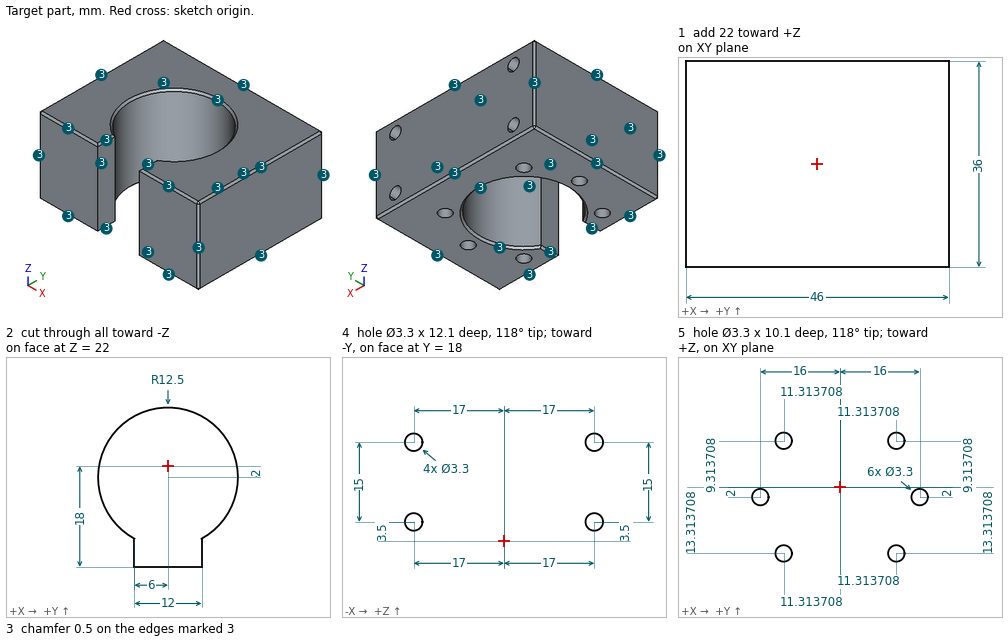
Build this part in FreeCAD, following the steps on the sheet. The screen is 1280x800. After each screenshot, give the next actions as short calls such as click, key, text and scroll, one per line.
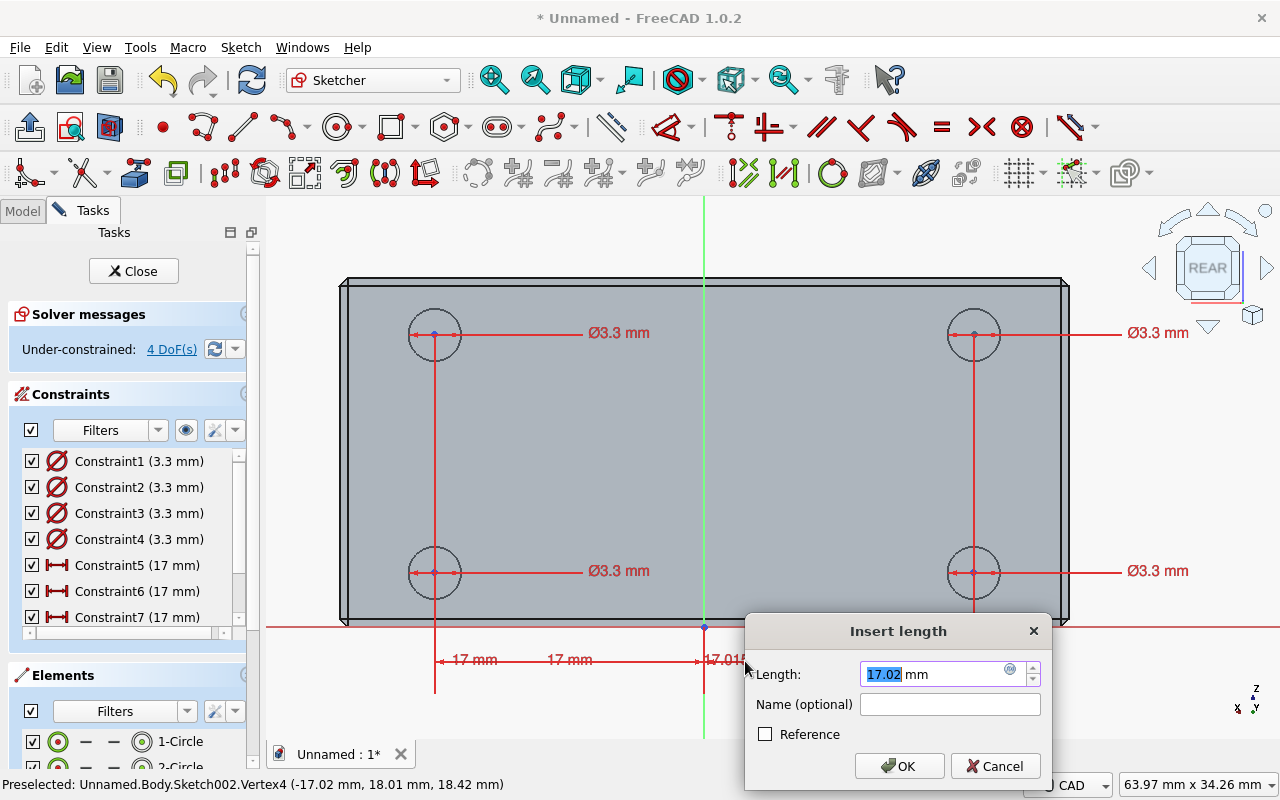
text(17)
key(Return)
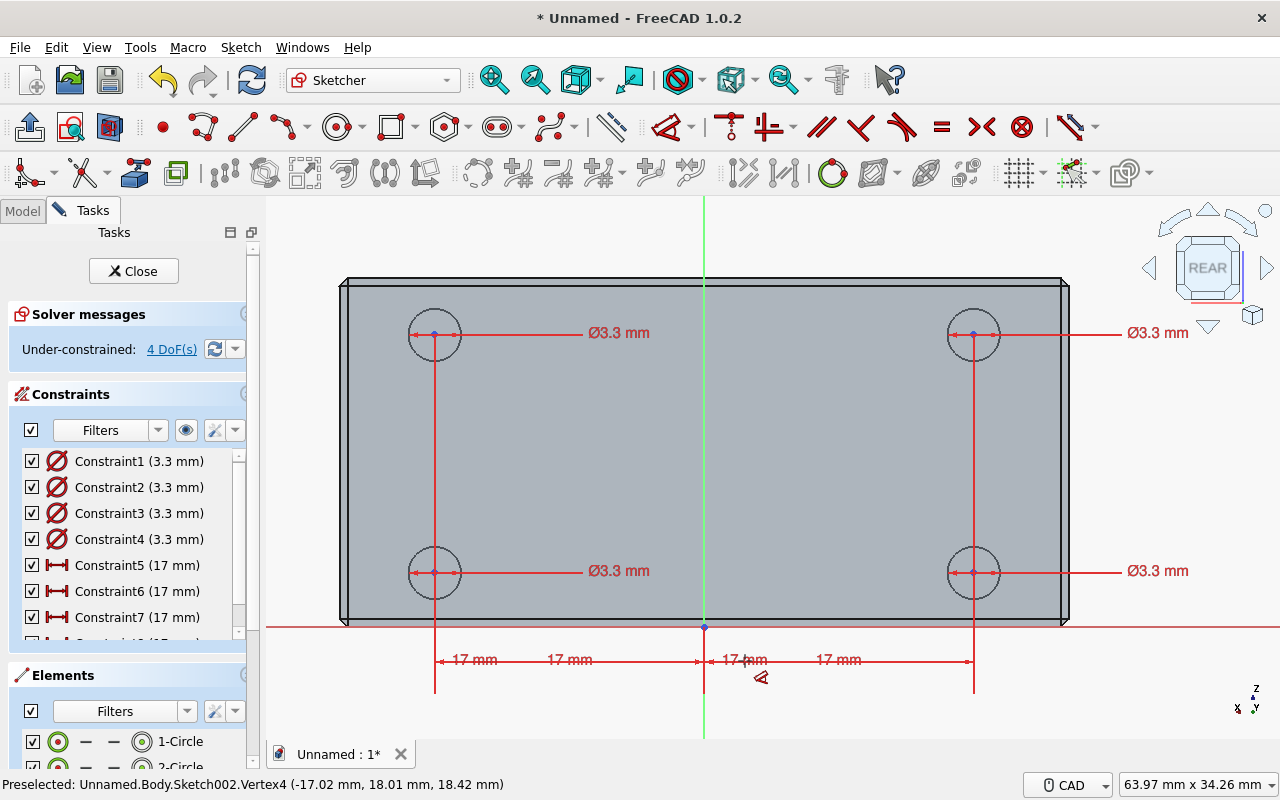
click(435, 573)
click(401, 600)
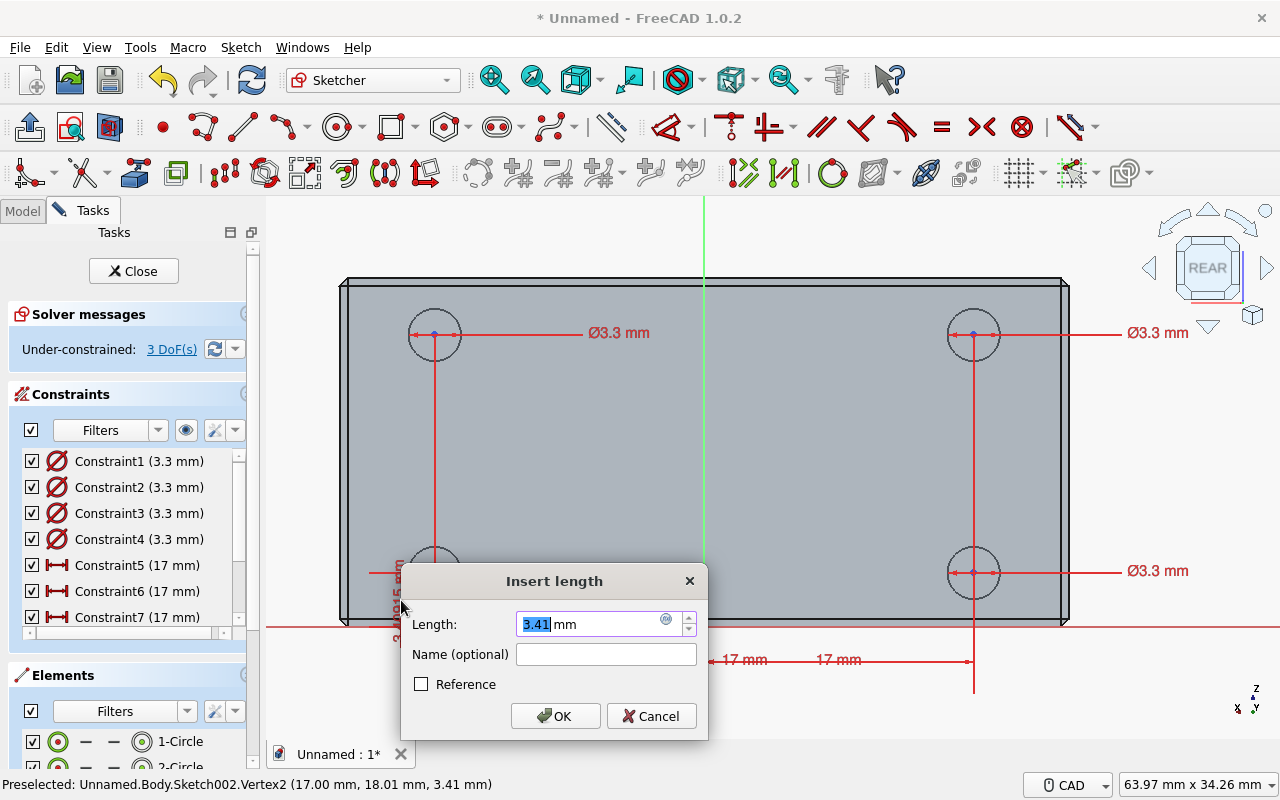
text(3.5)
key(Return)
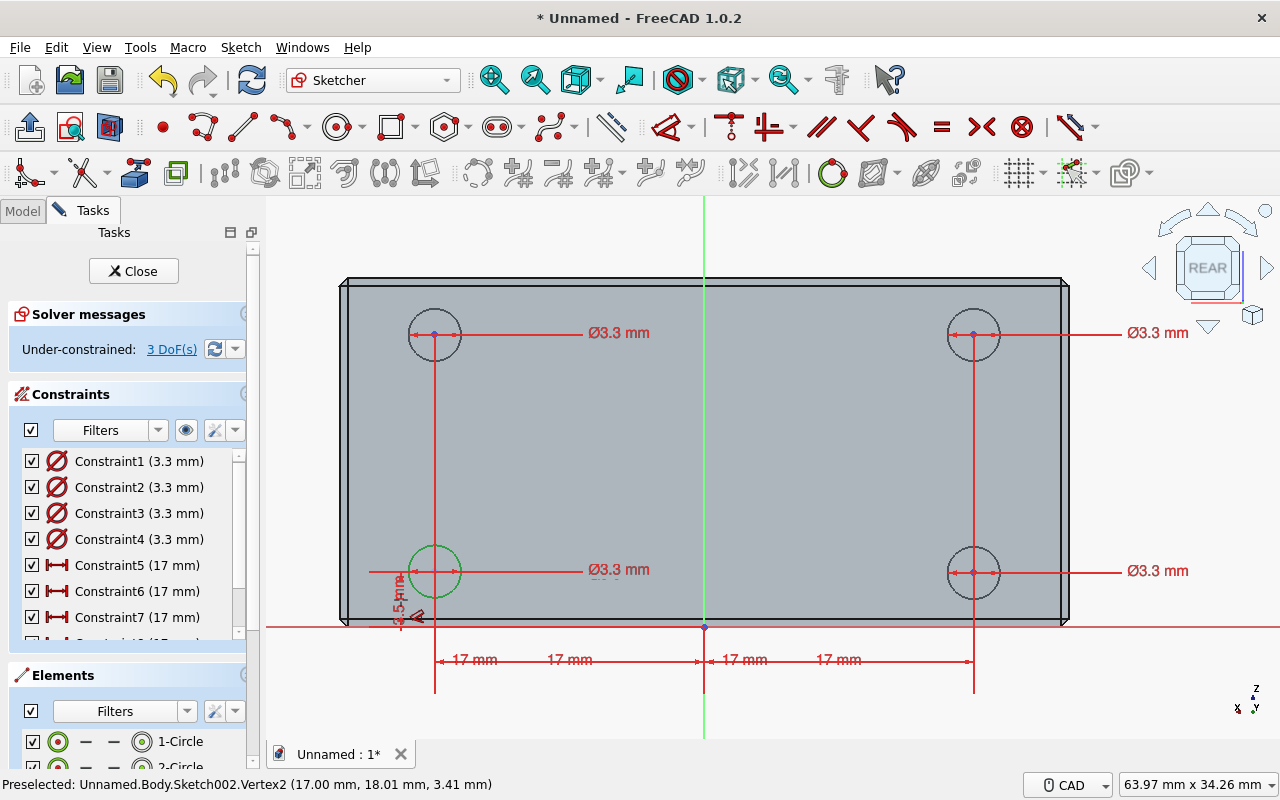
click(974, 573)
click(1008, 600)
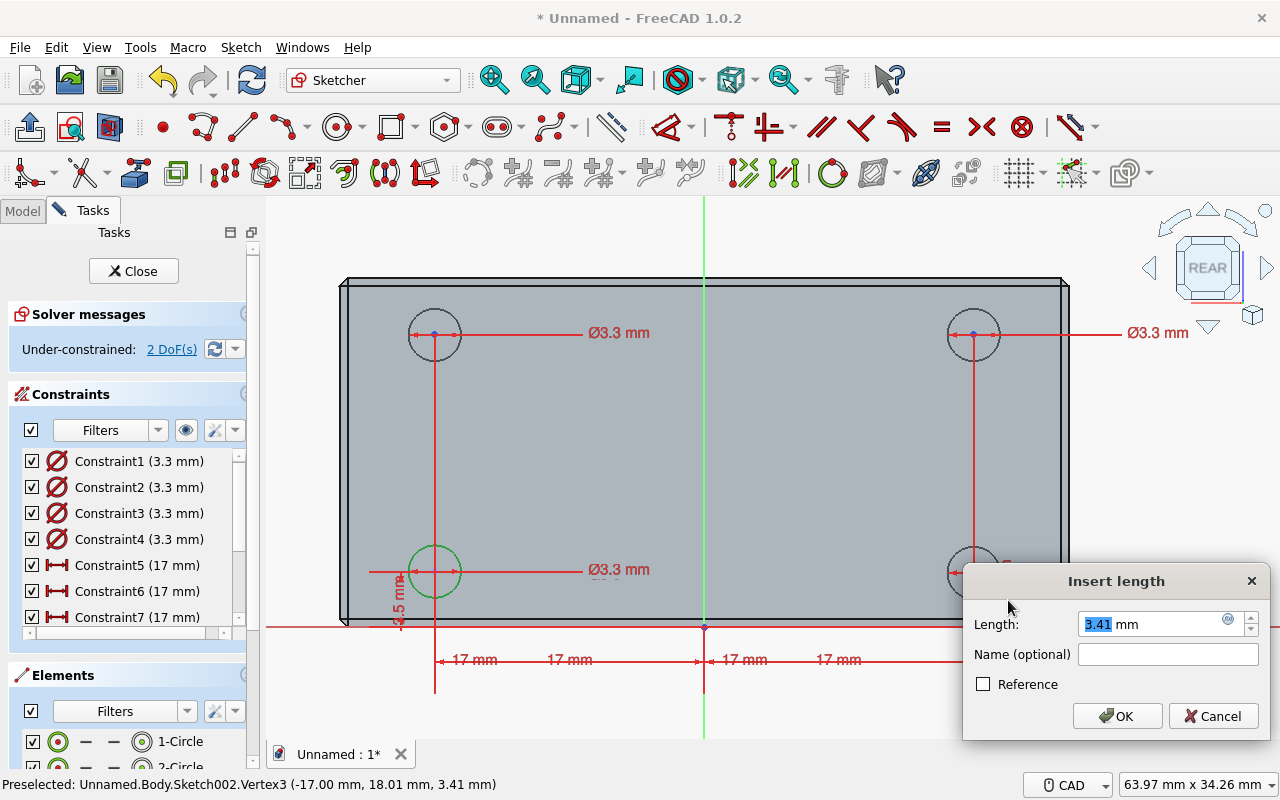
text(3.5)
key(Return)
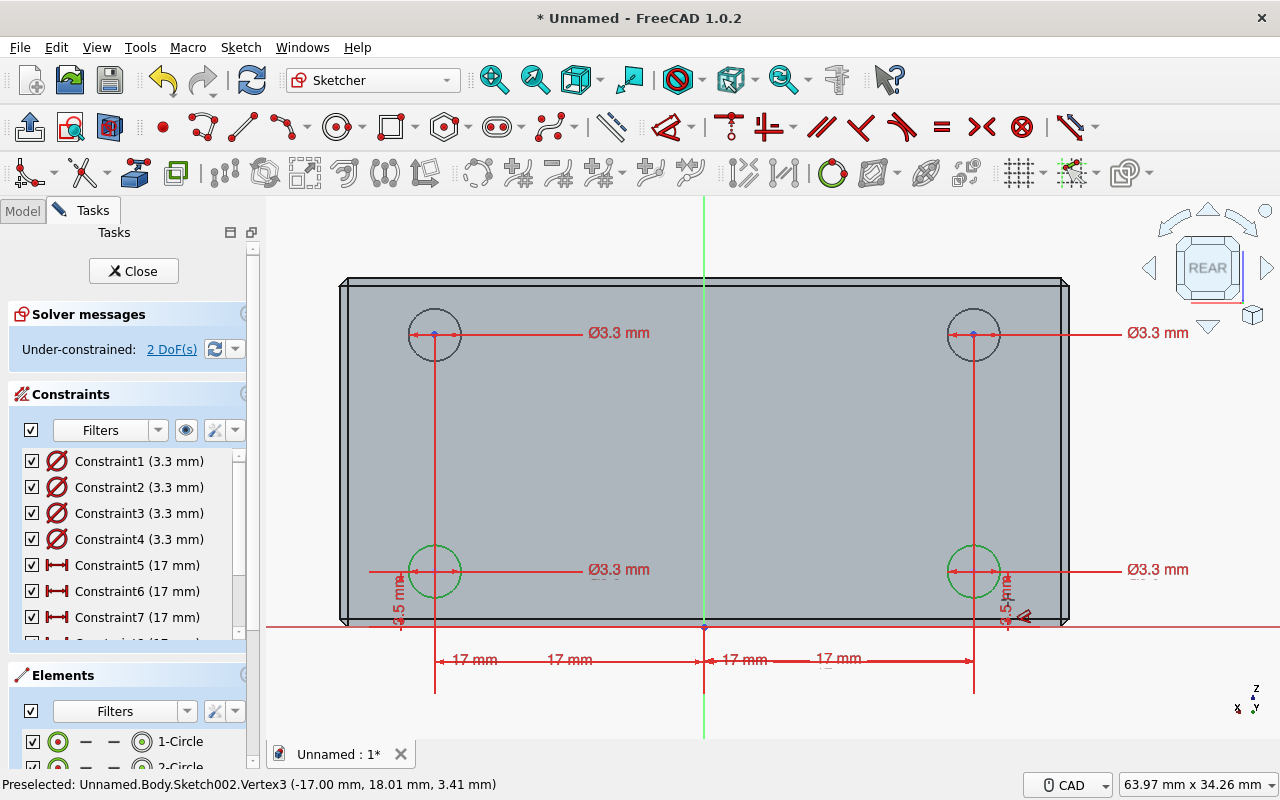
click(435, 335)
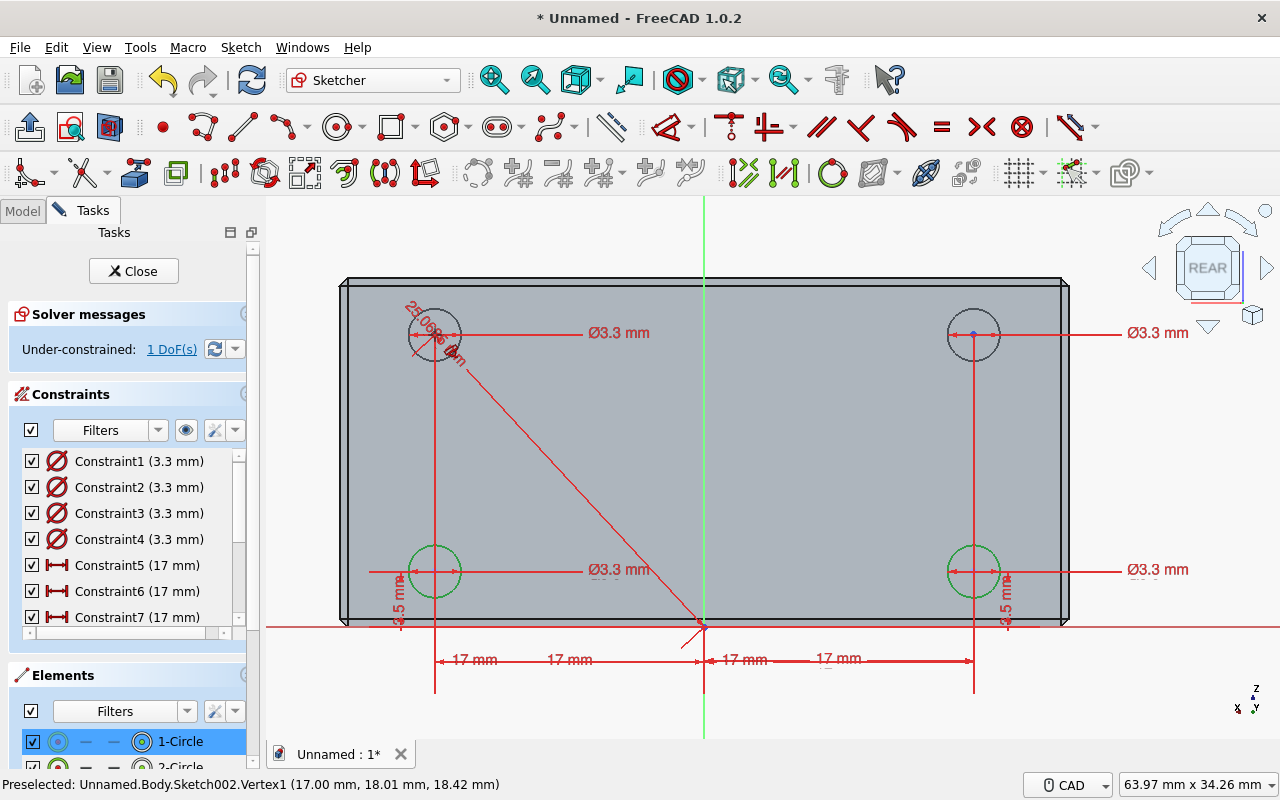
click(435, 572)
click(401, 453)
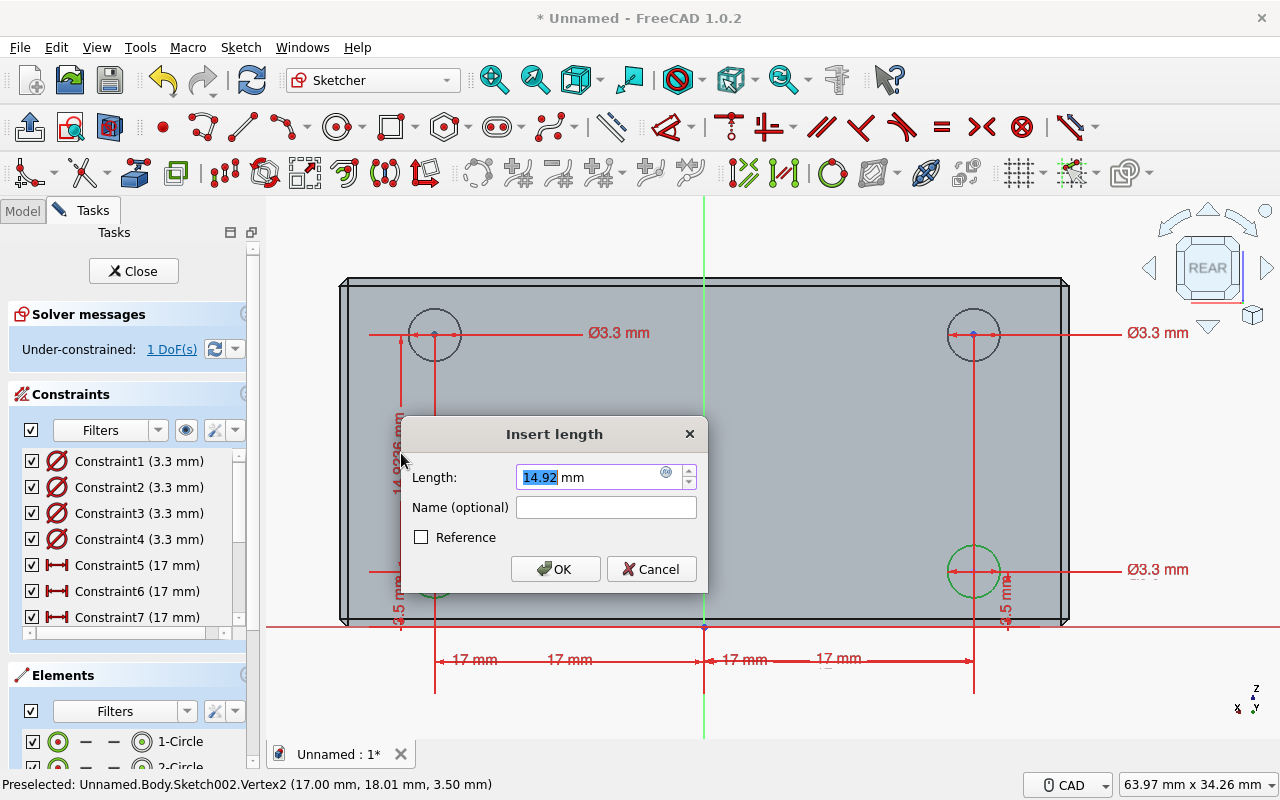
text(15)
key(Return)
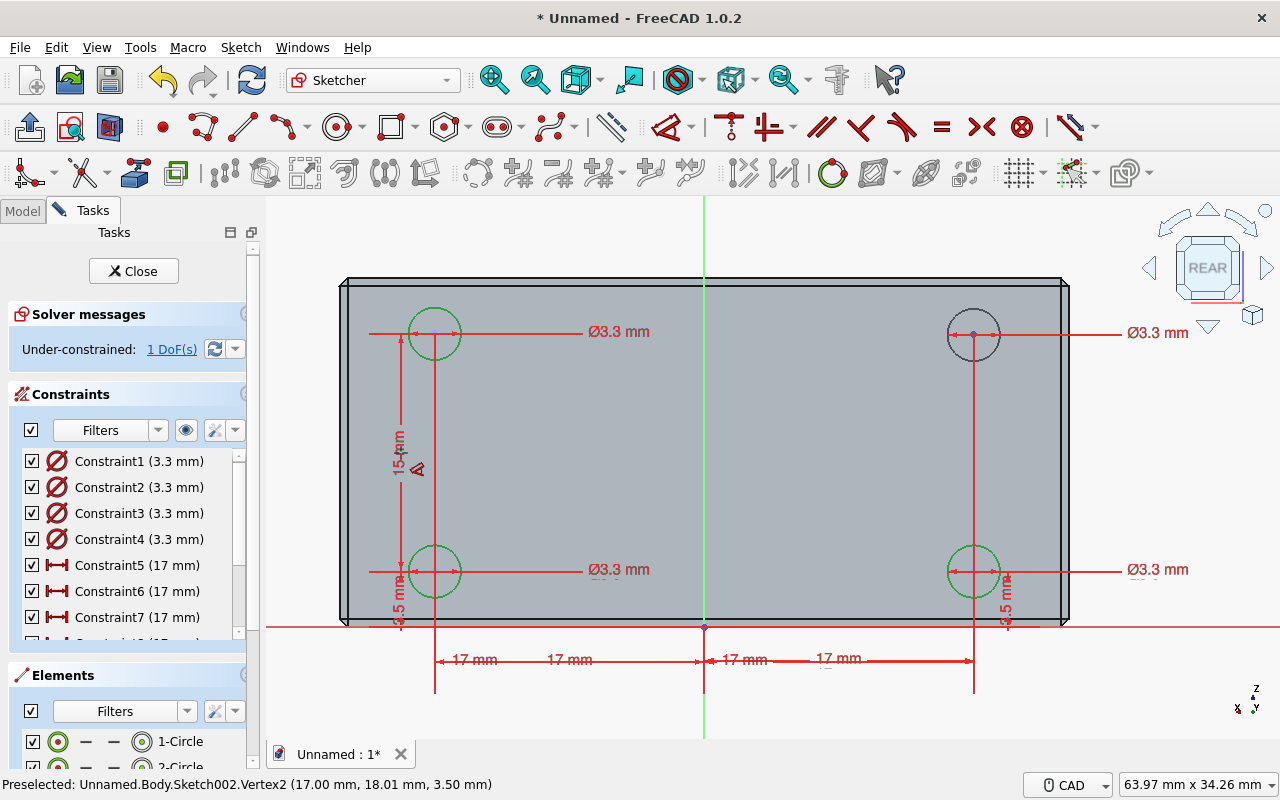
click(974, 572)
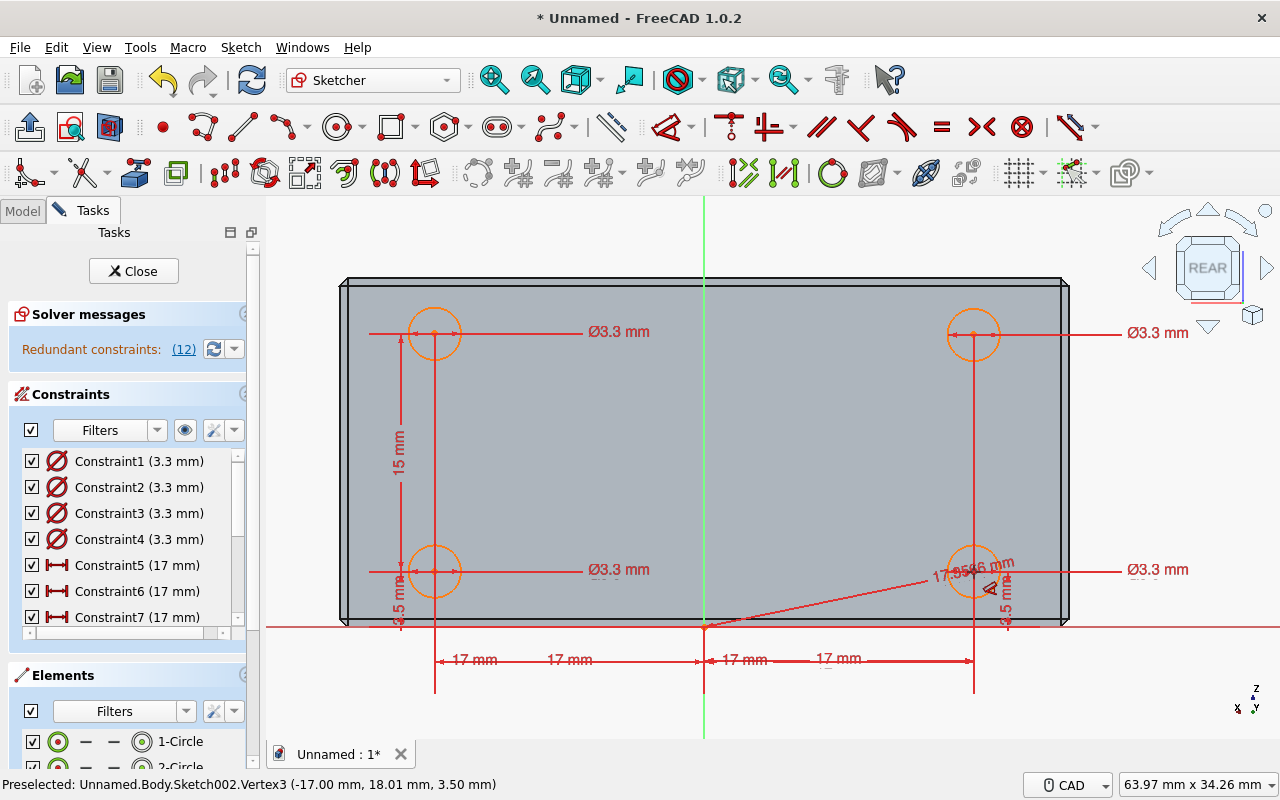
click(974, 335)
click(1008, 453)